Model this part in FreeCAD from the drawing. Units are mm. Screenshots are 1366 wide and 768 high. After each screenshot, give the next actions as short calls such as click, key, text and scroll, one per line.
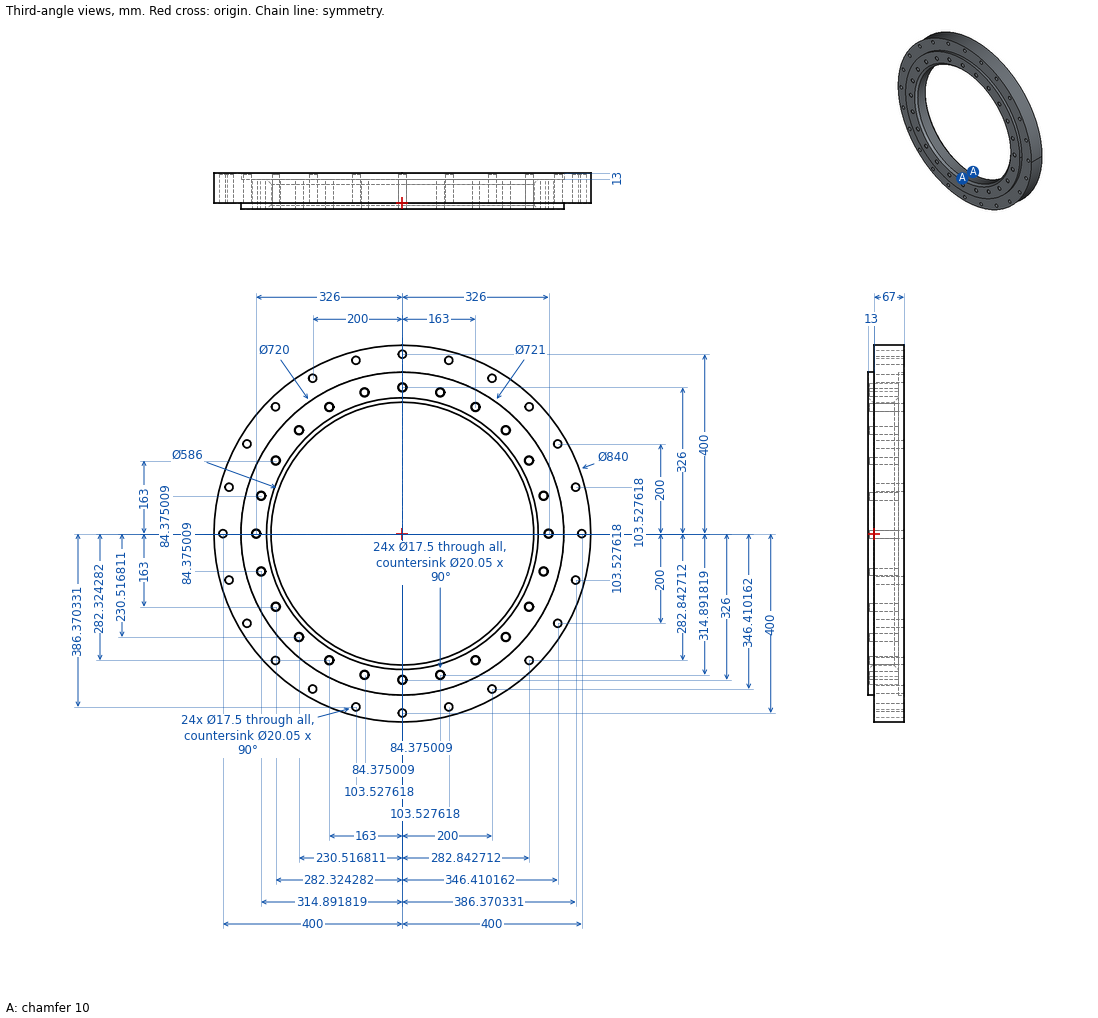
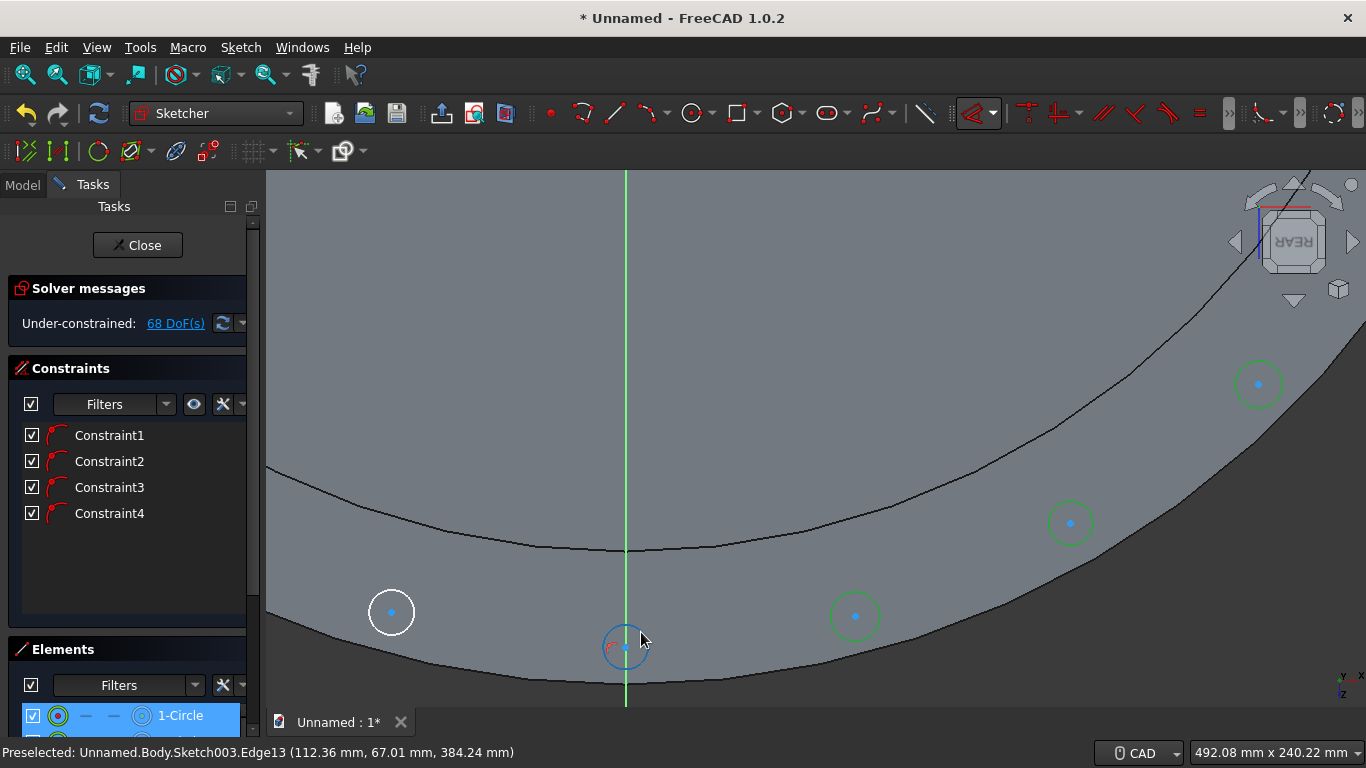
click(641, 631)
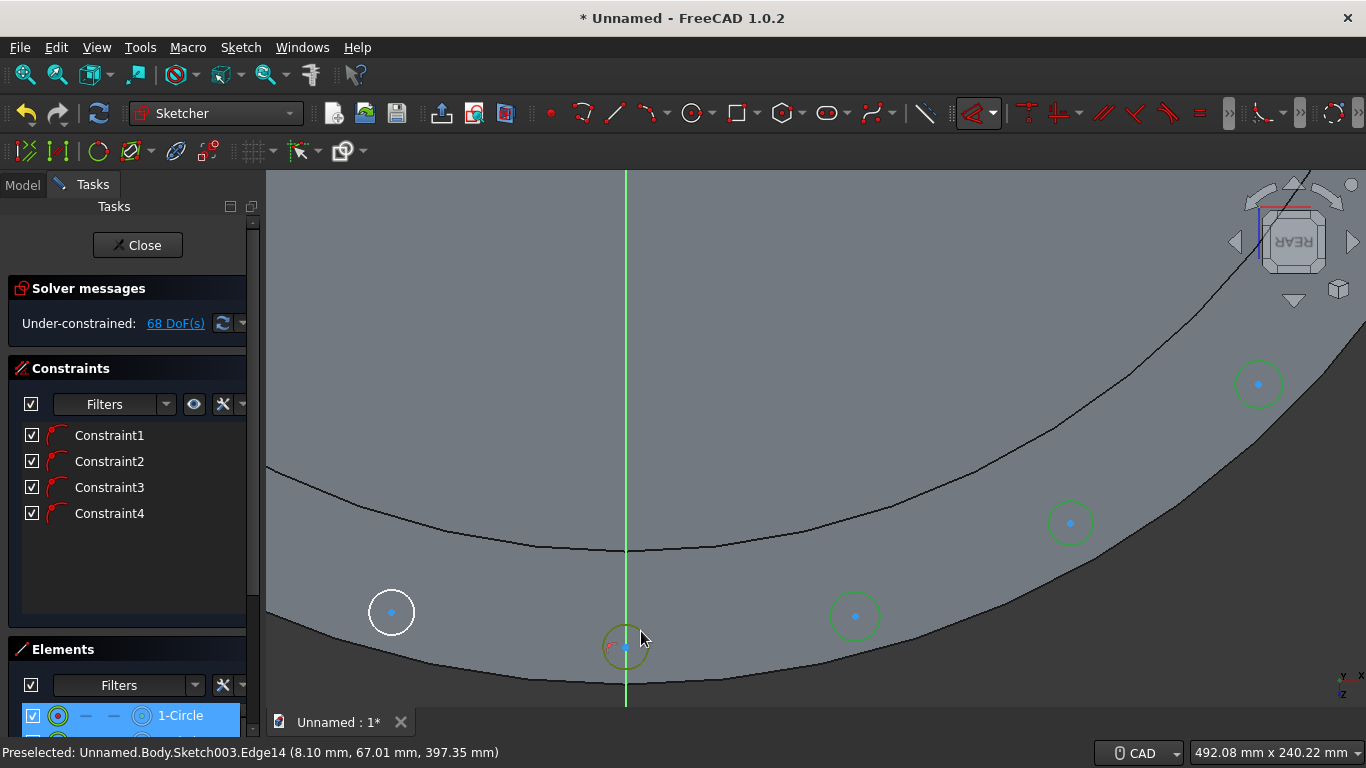
click(408, 597)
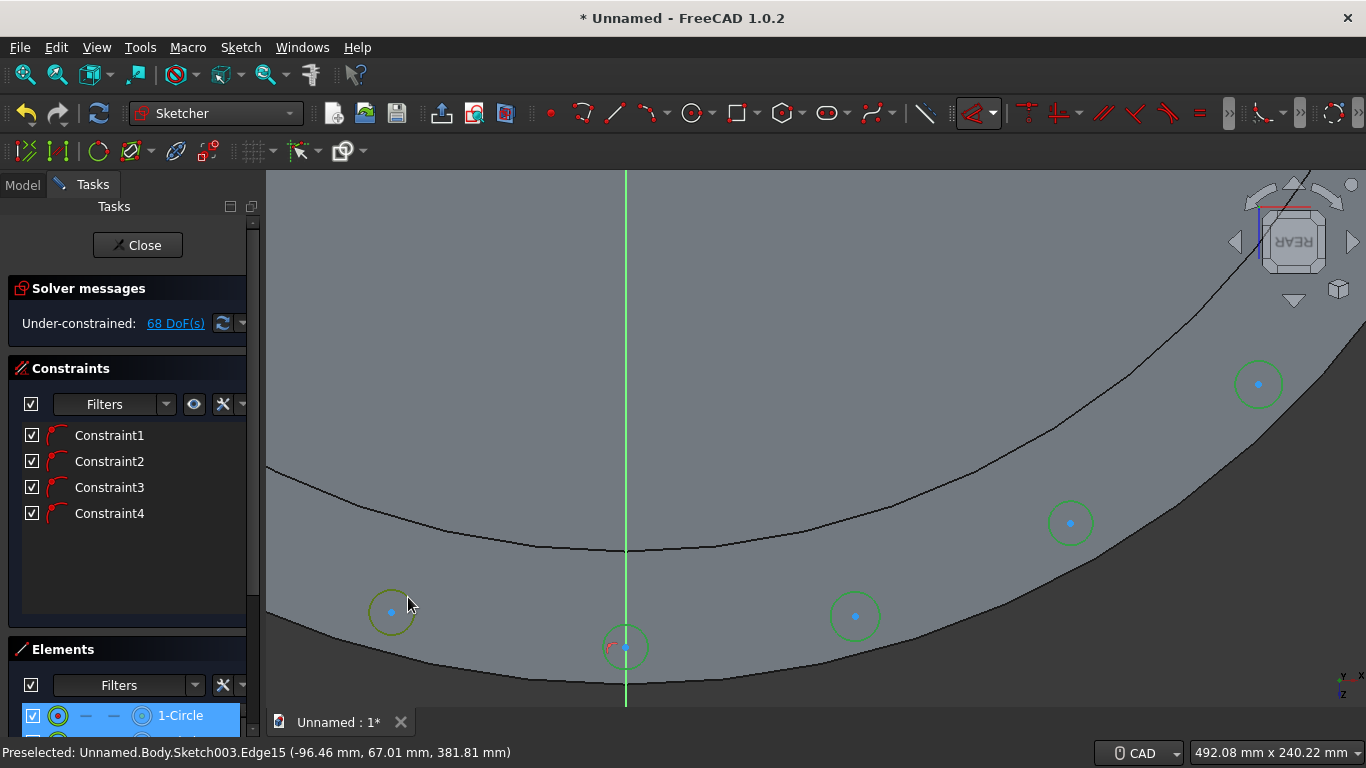
scroll(778, 614, down, 8)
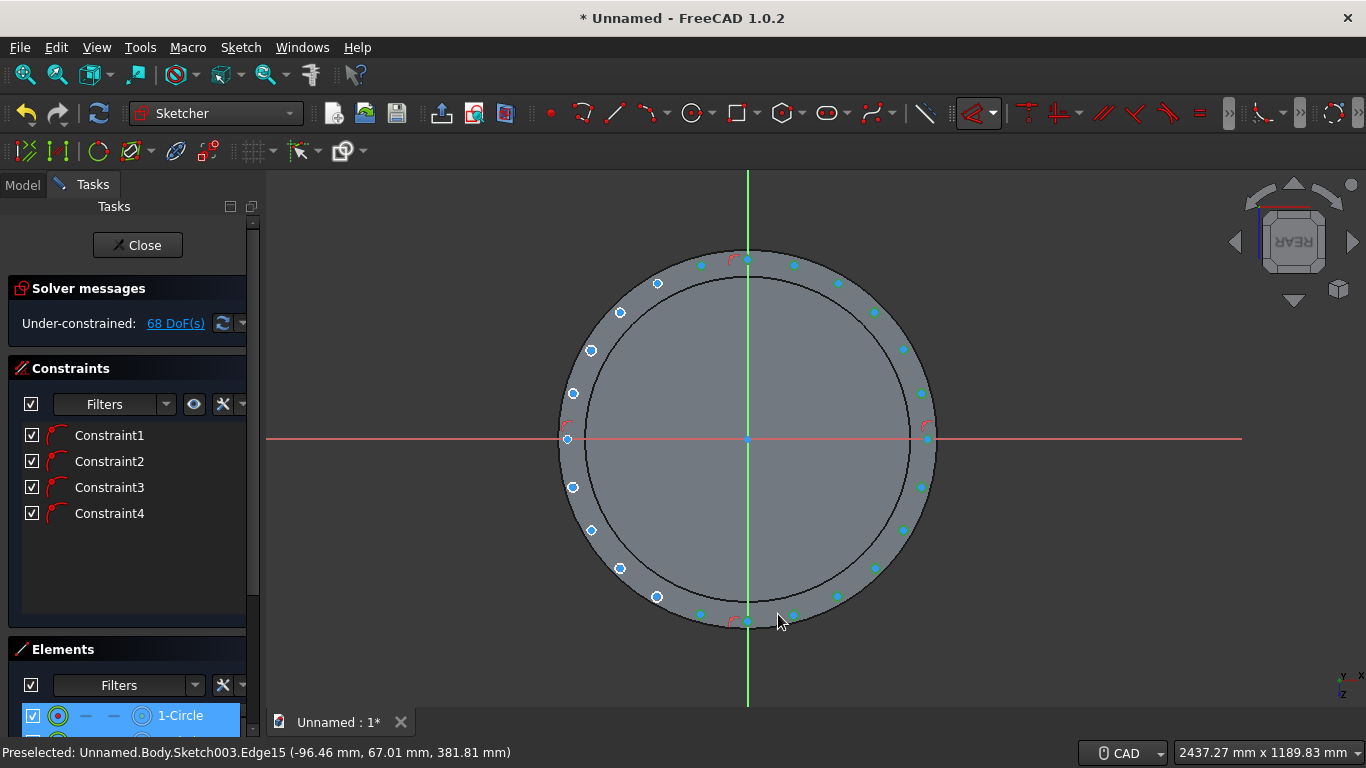
scroll(661, 593, up, 5)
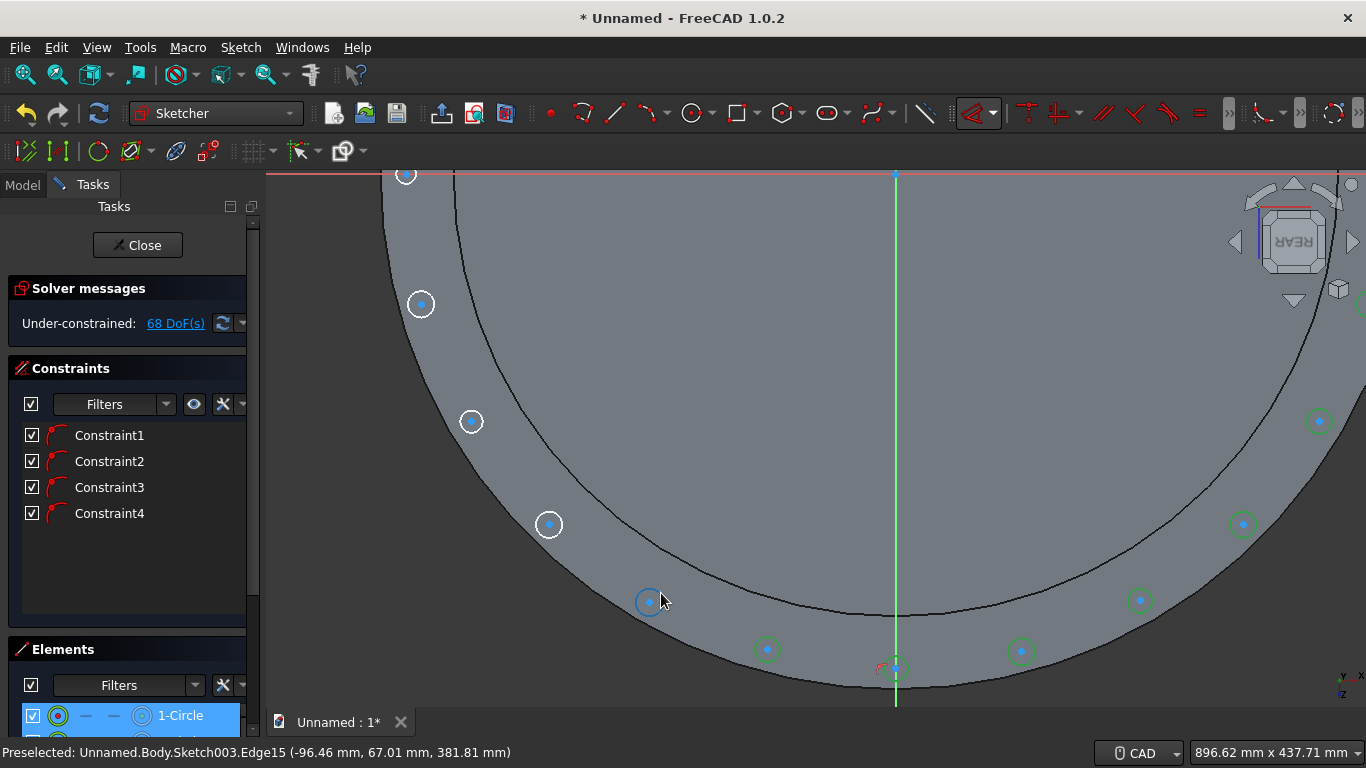
click(659, 593)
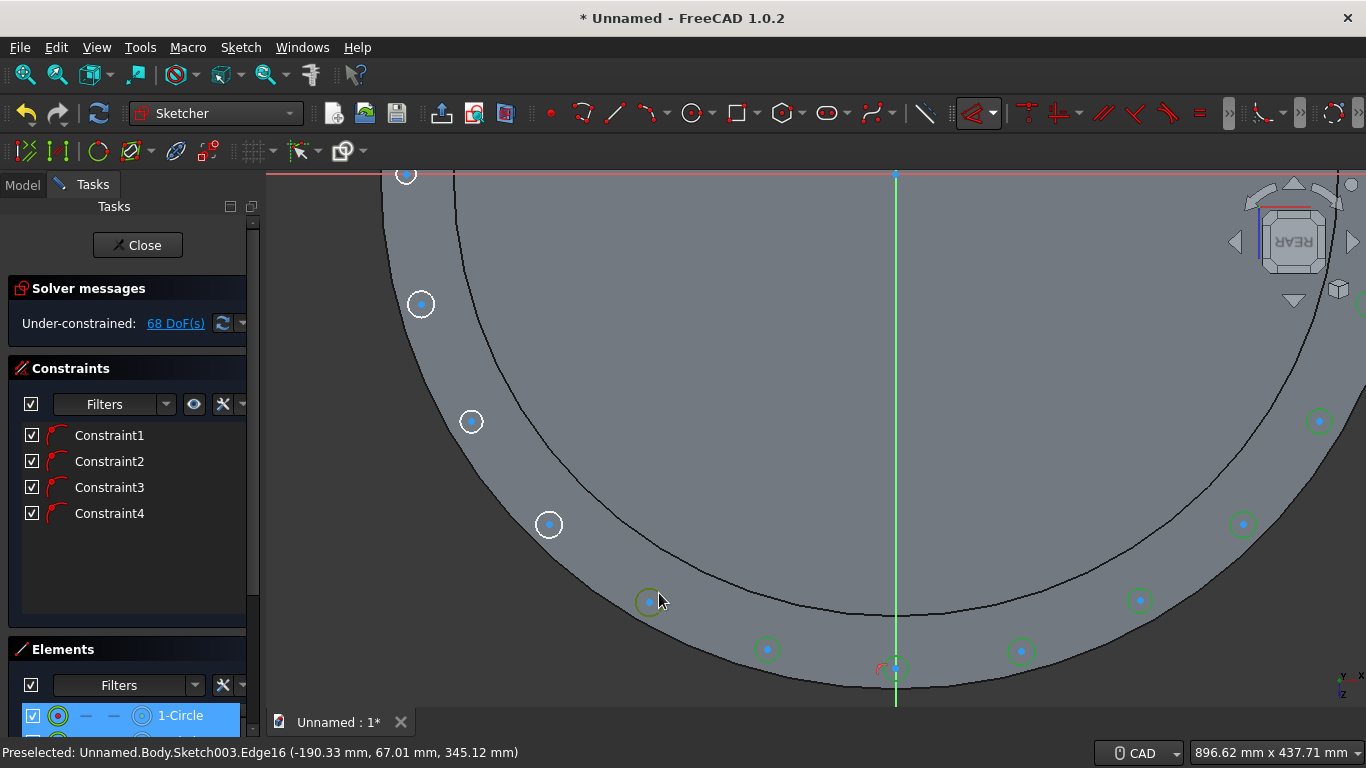
click(558, 516)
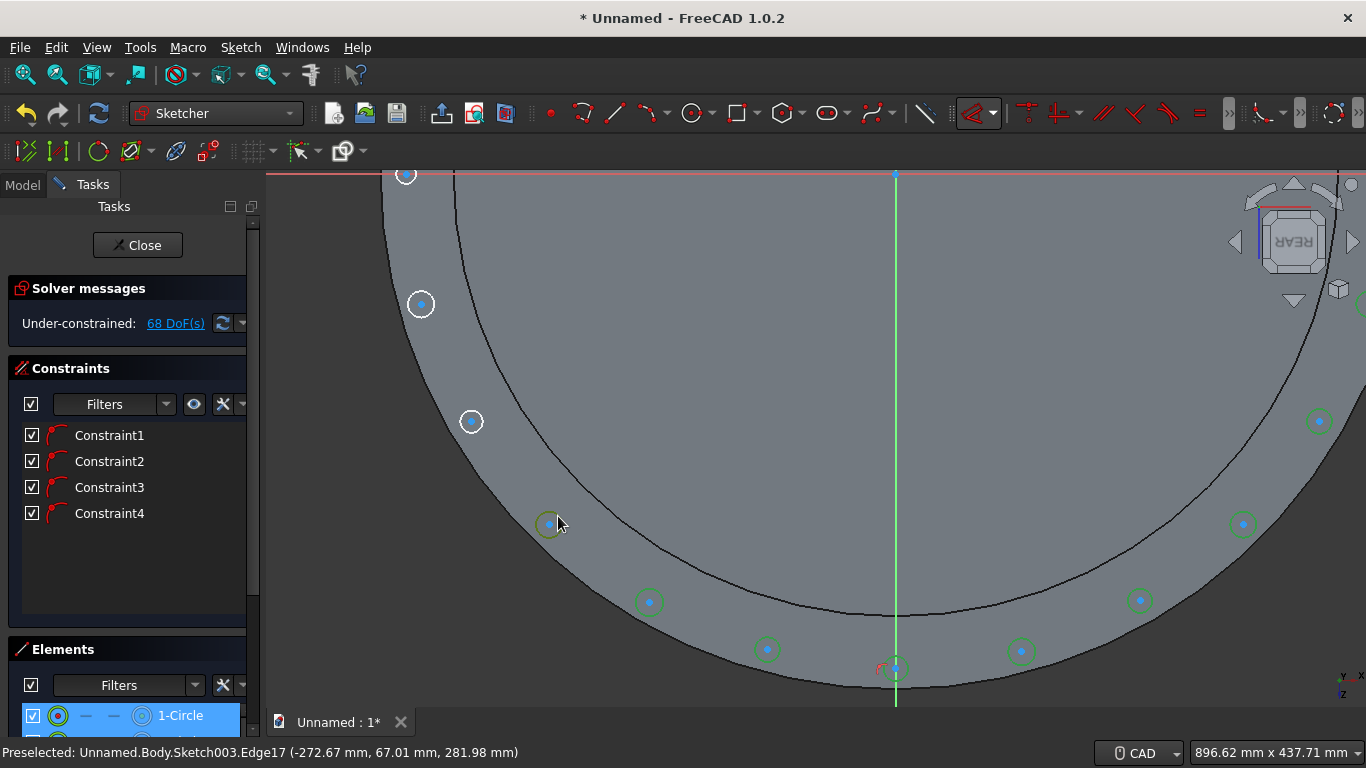
scroll(479, 414, up, 2)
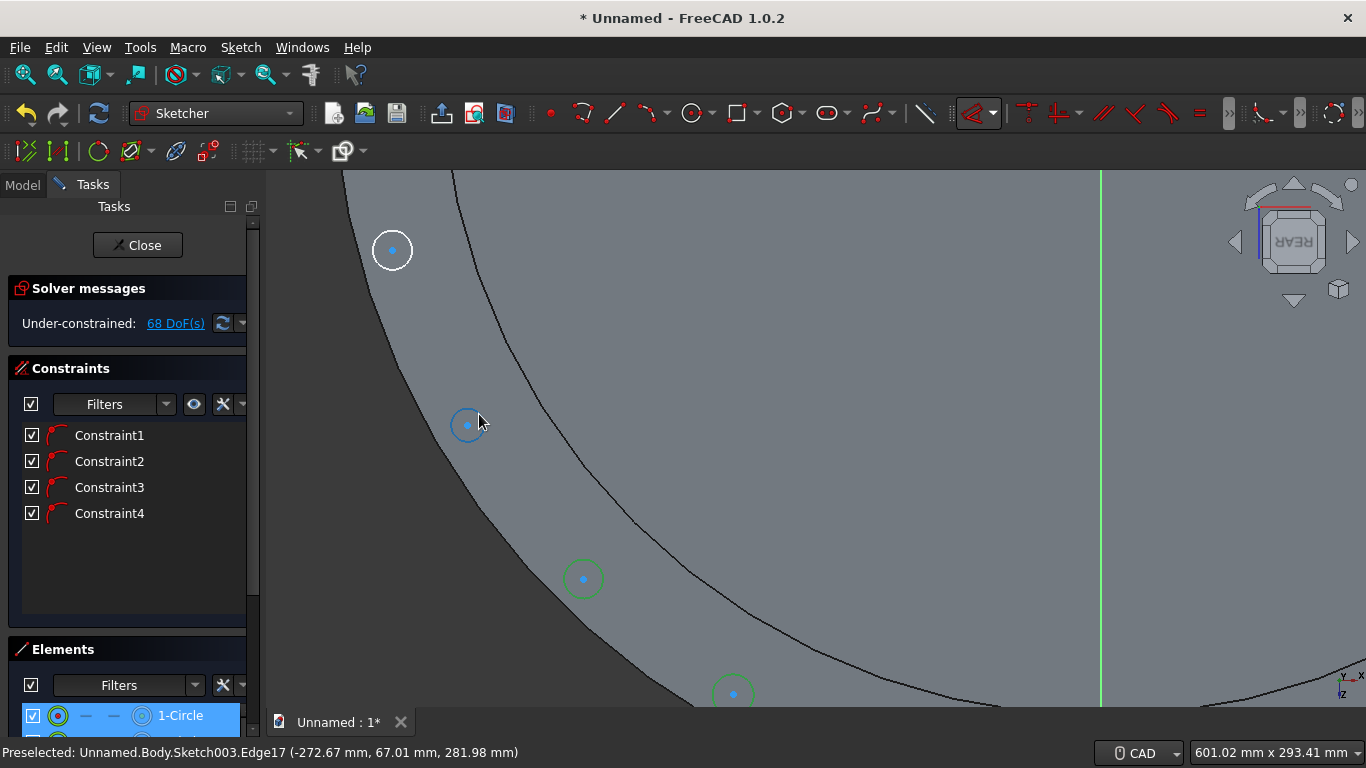
click(479, 413)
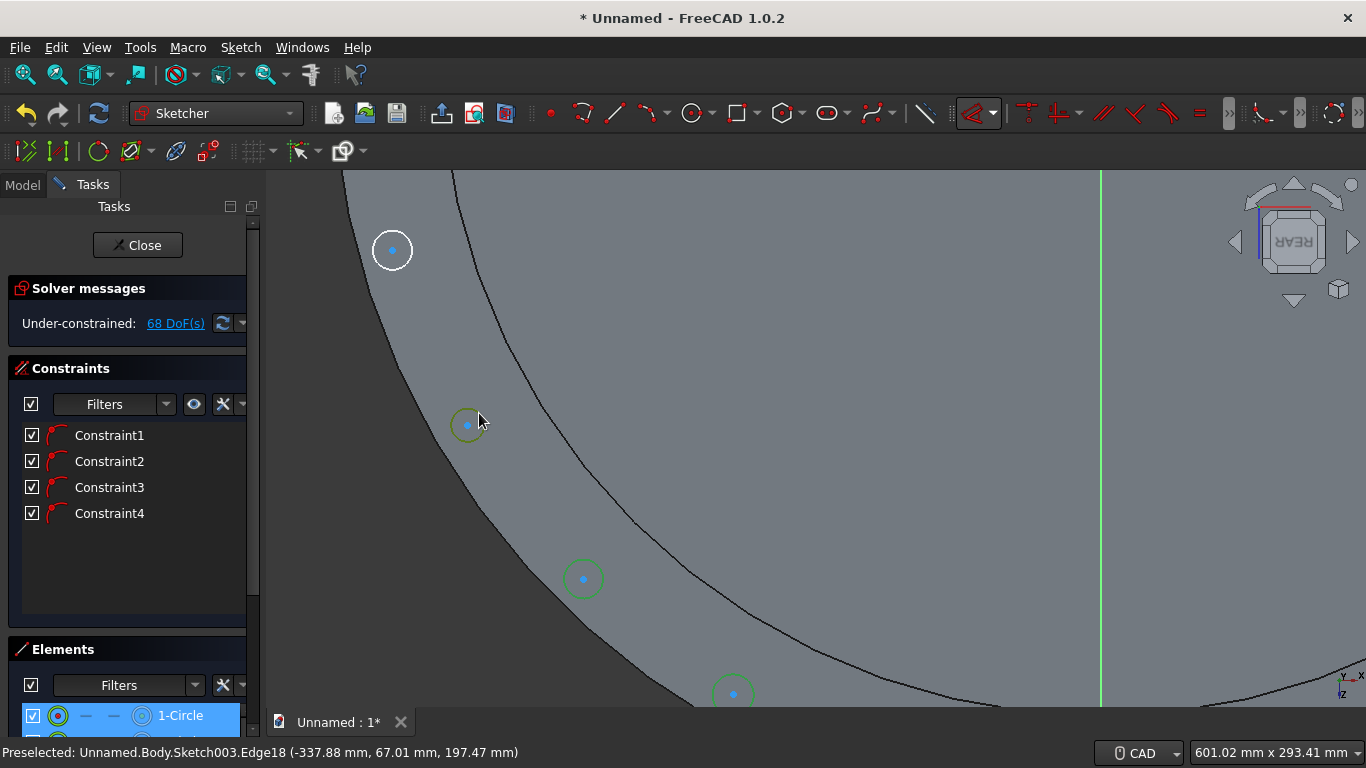
click(406, 236)